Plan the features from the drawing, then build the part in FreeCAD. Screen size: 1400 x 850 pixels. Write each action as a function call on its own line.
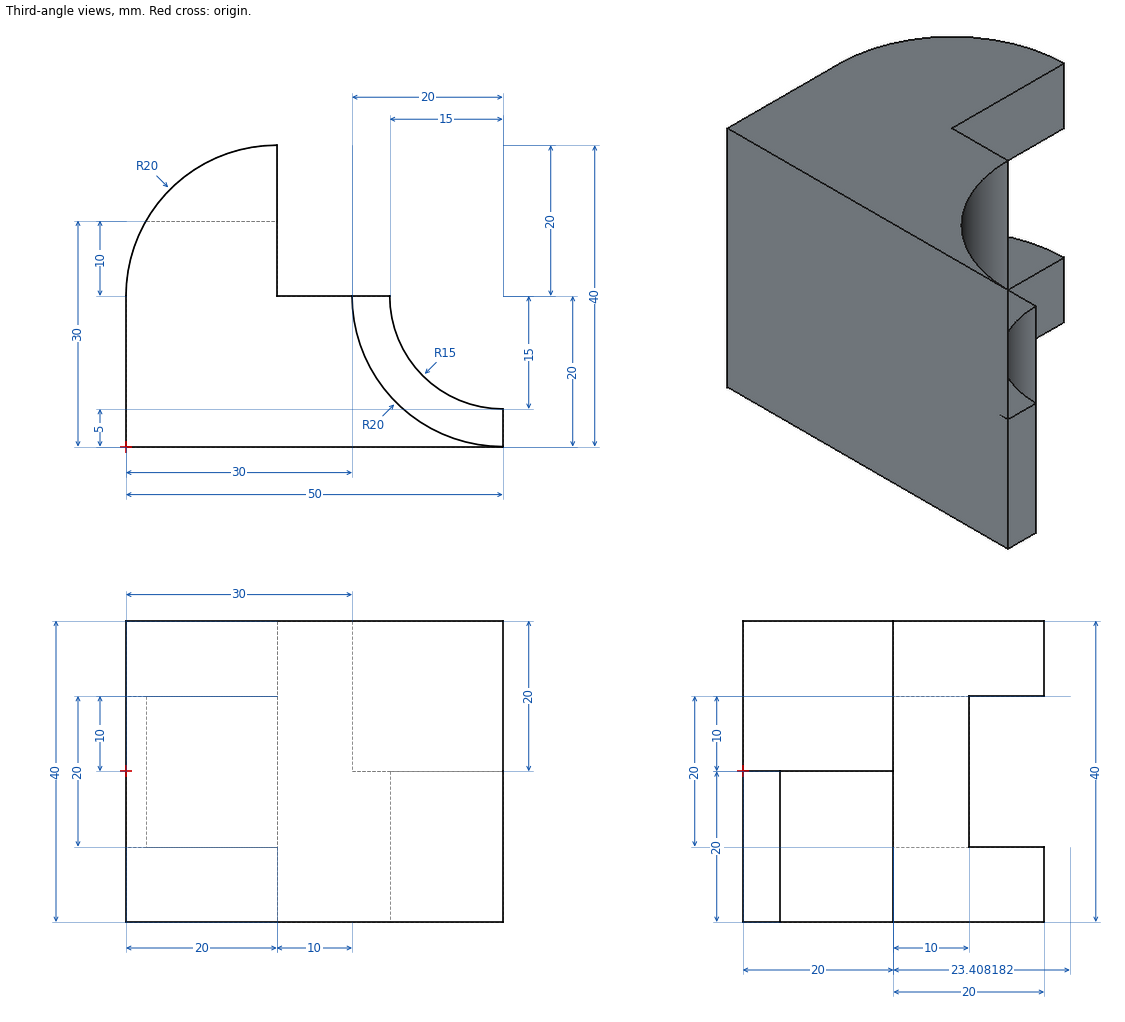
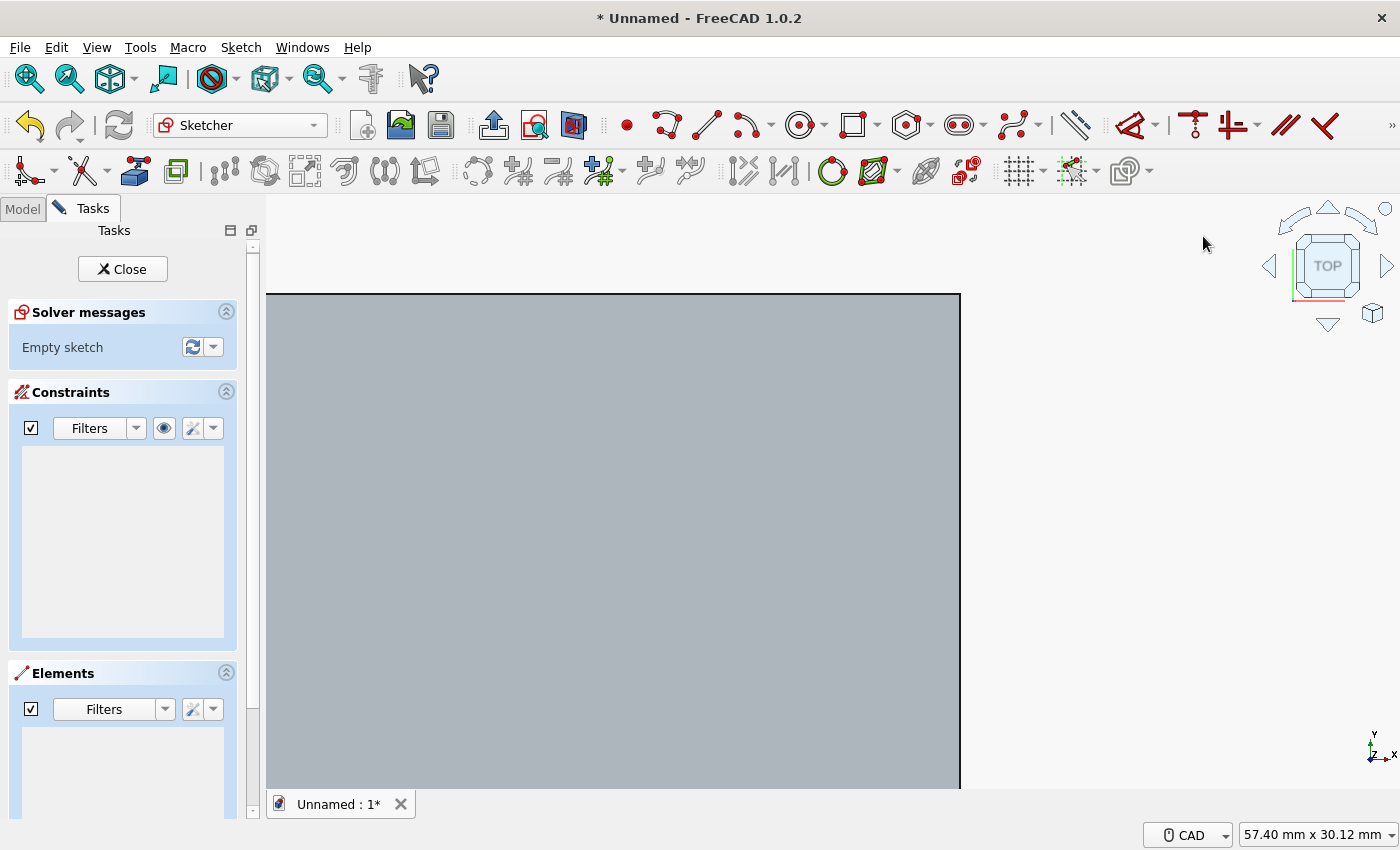
click(854, 126)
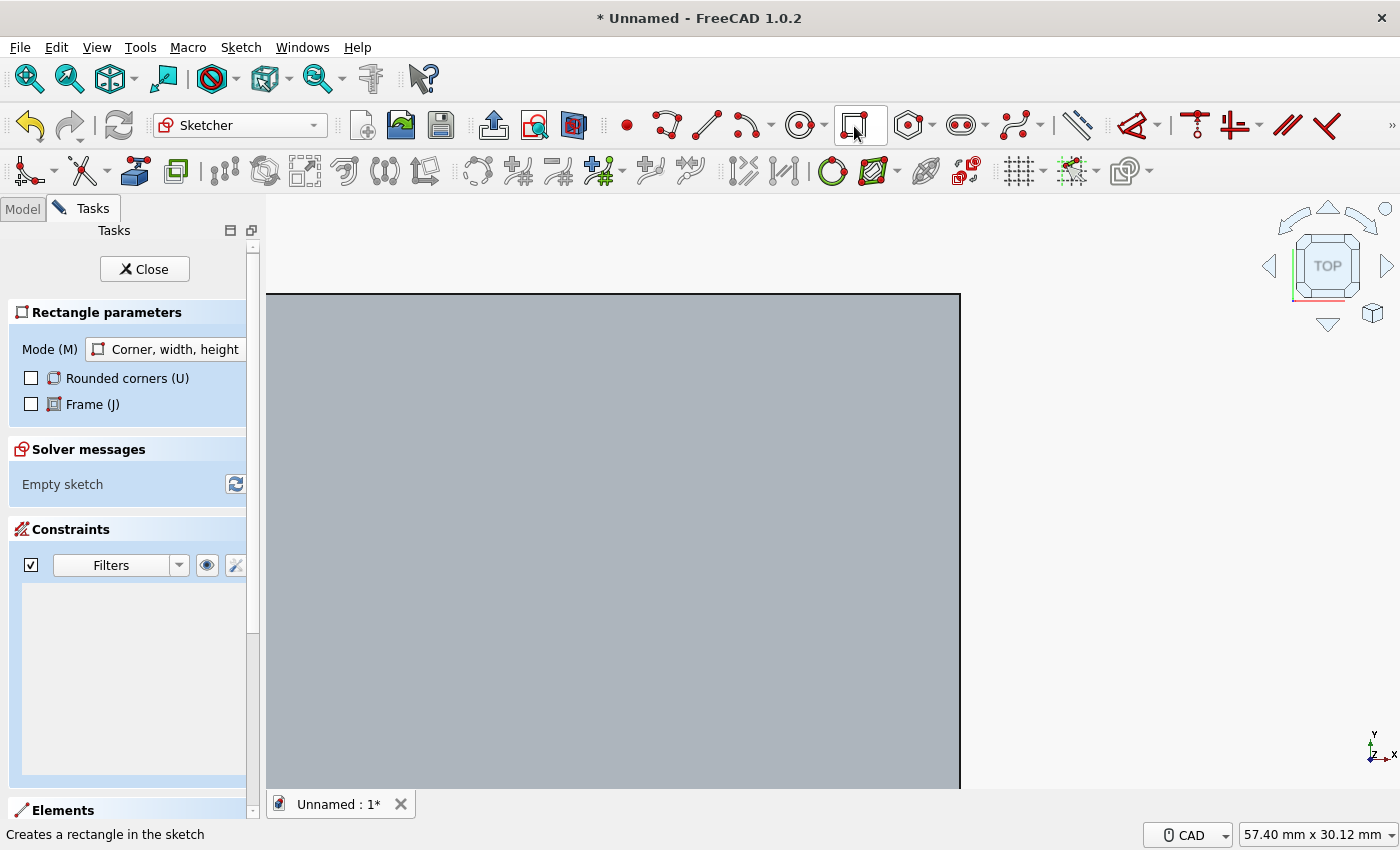
click(565, 294)
move(960, 689)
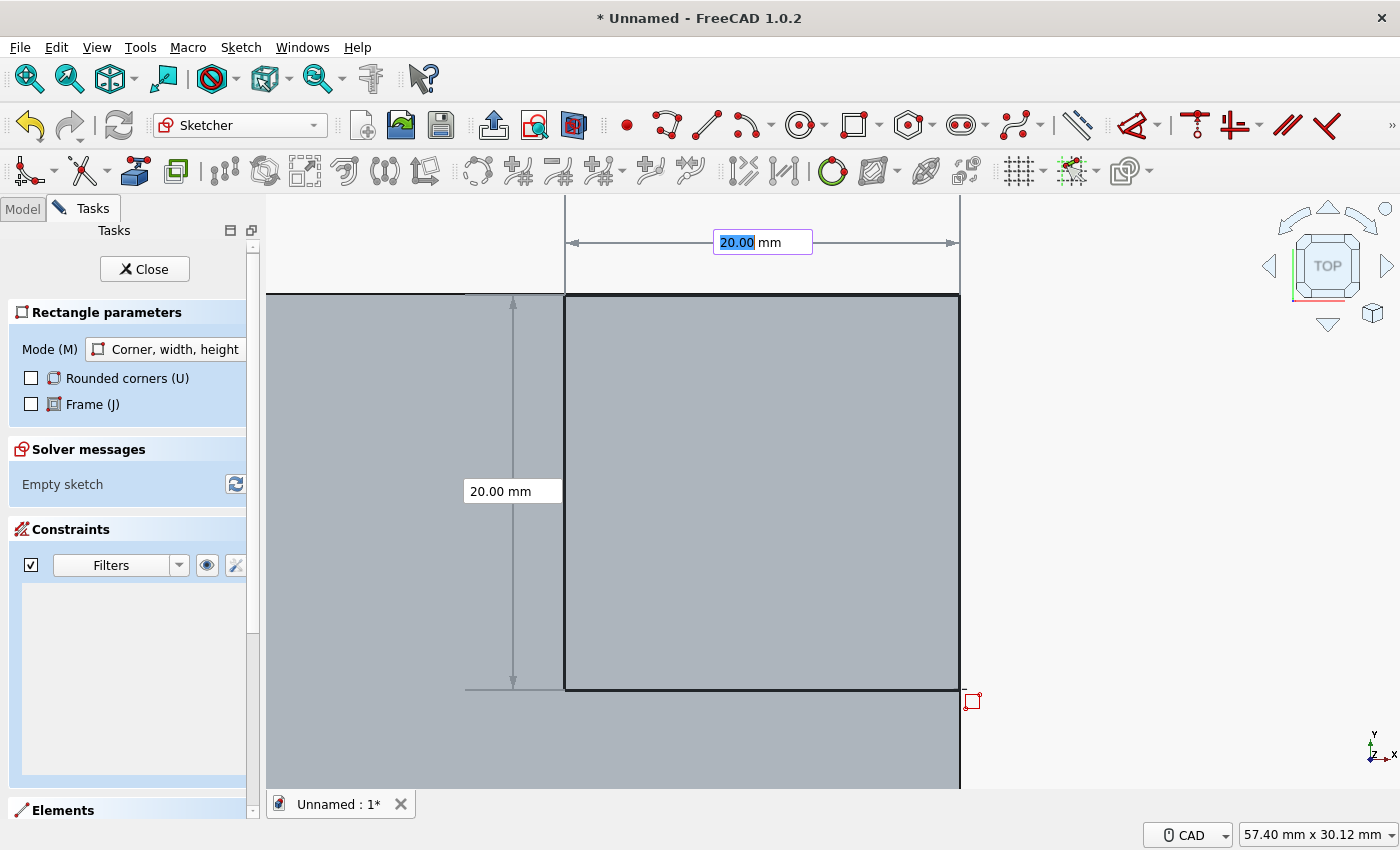
text(20)
key(Tab)
text(20)
key(Return)
key(Escape)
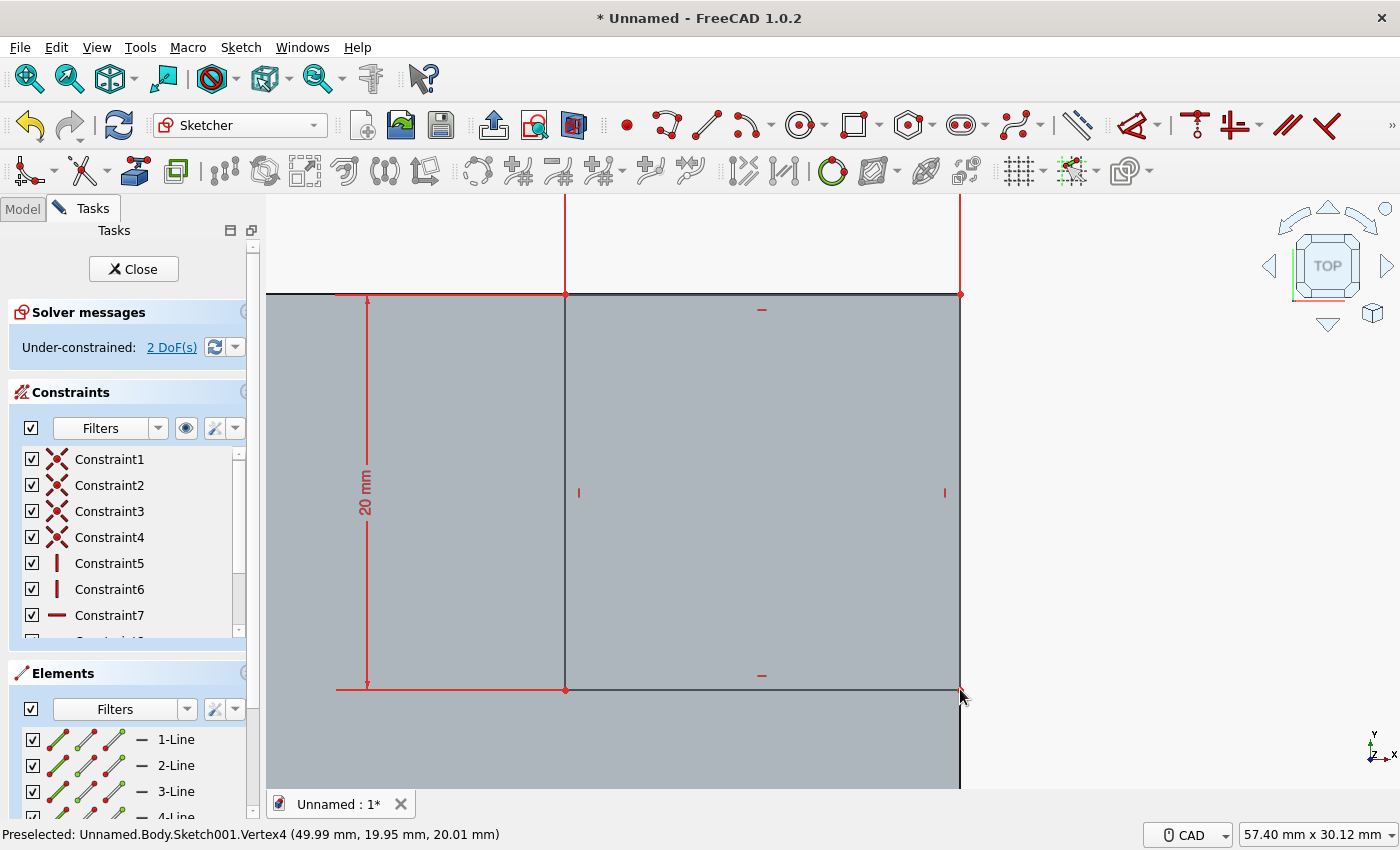
click(1132, 126)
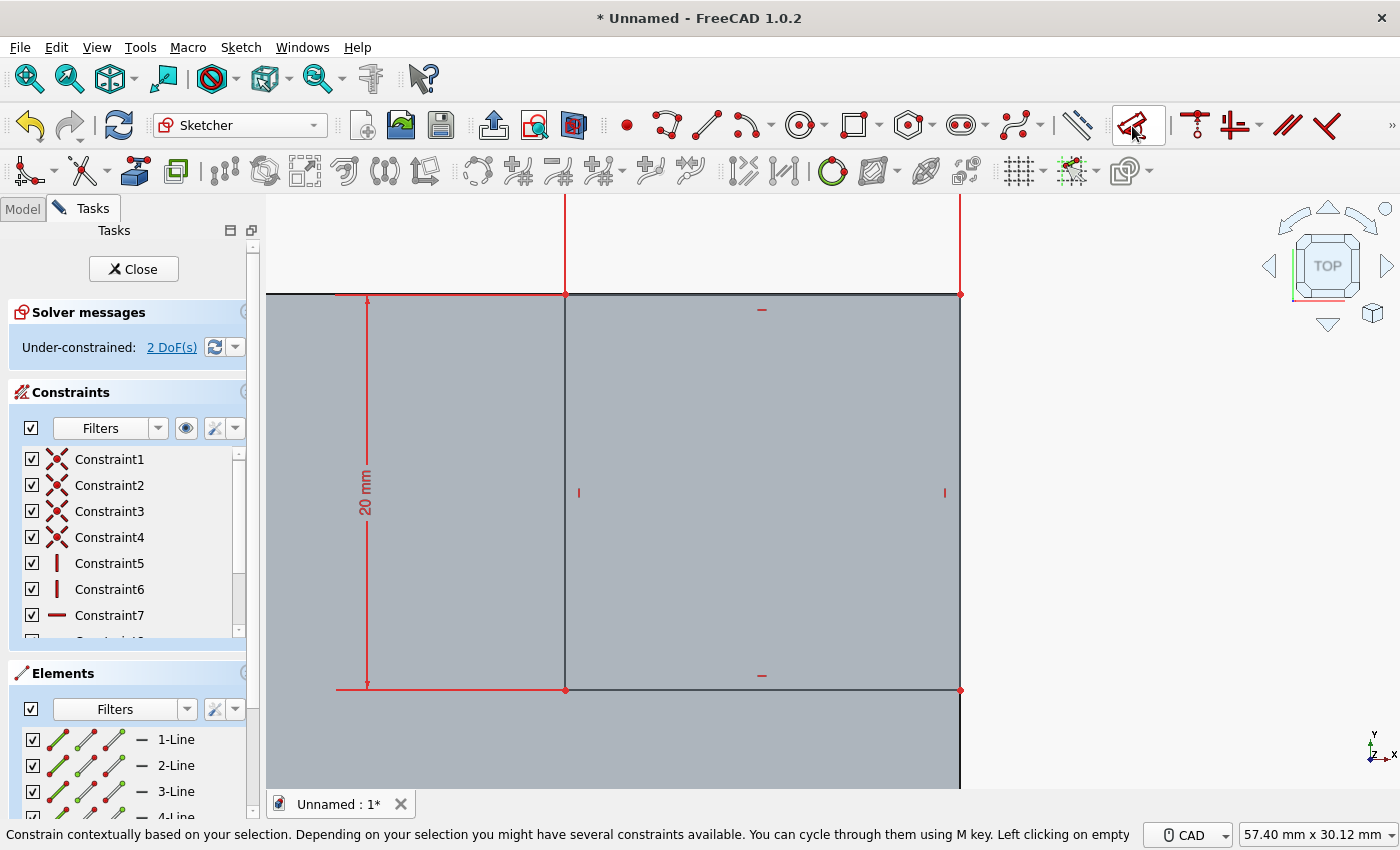
click(565, 295)
click(429, 261)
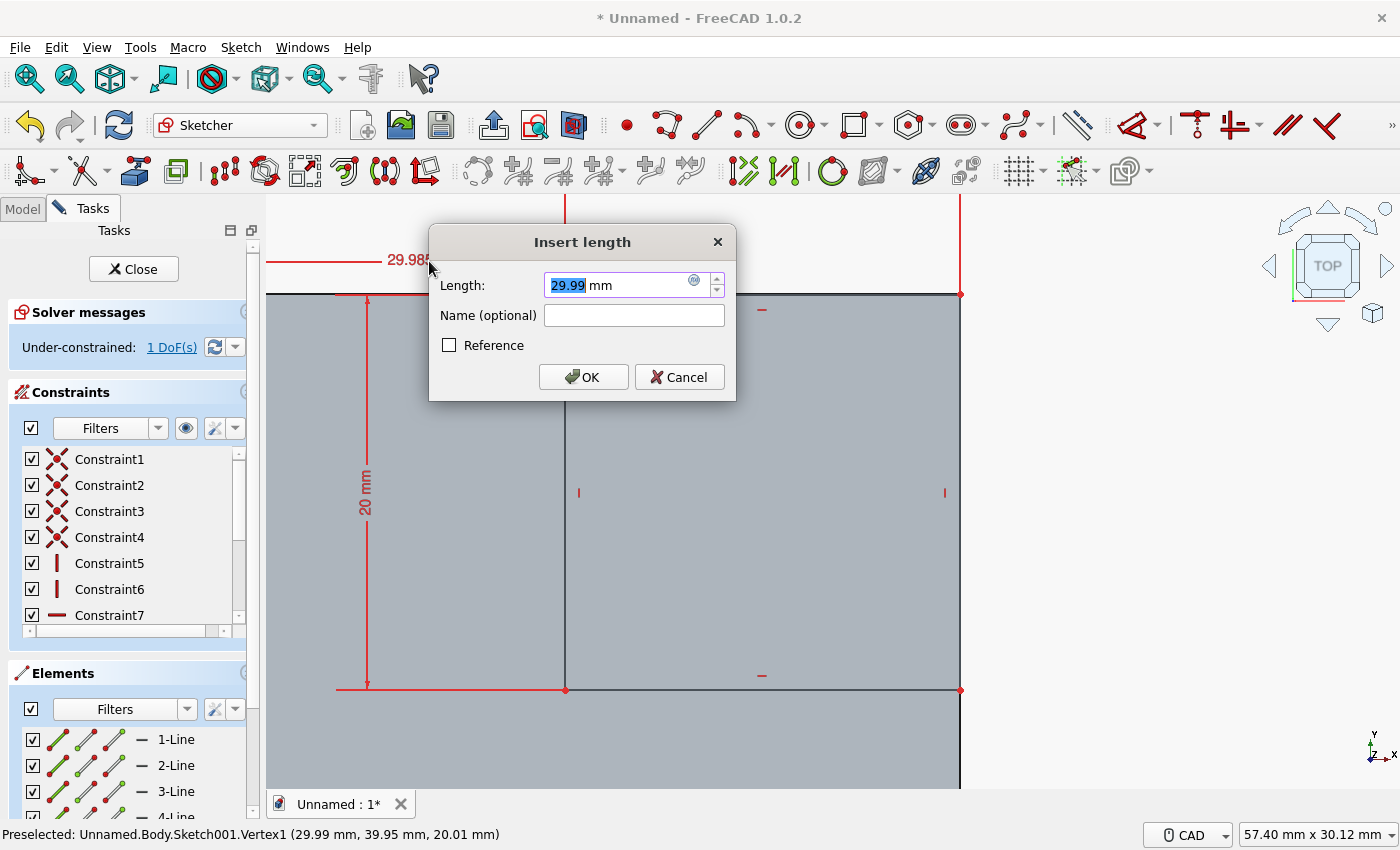
text(30)
key(Return)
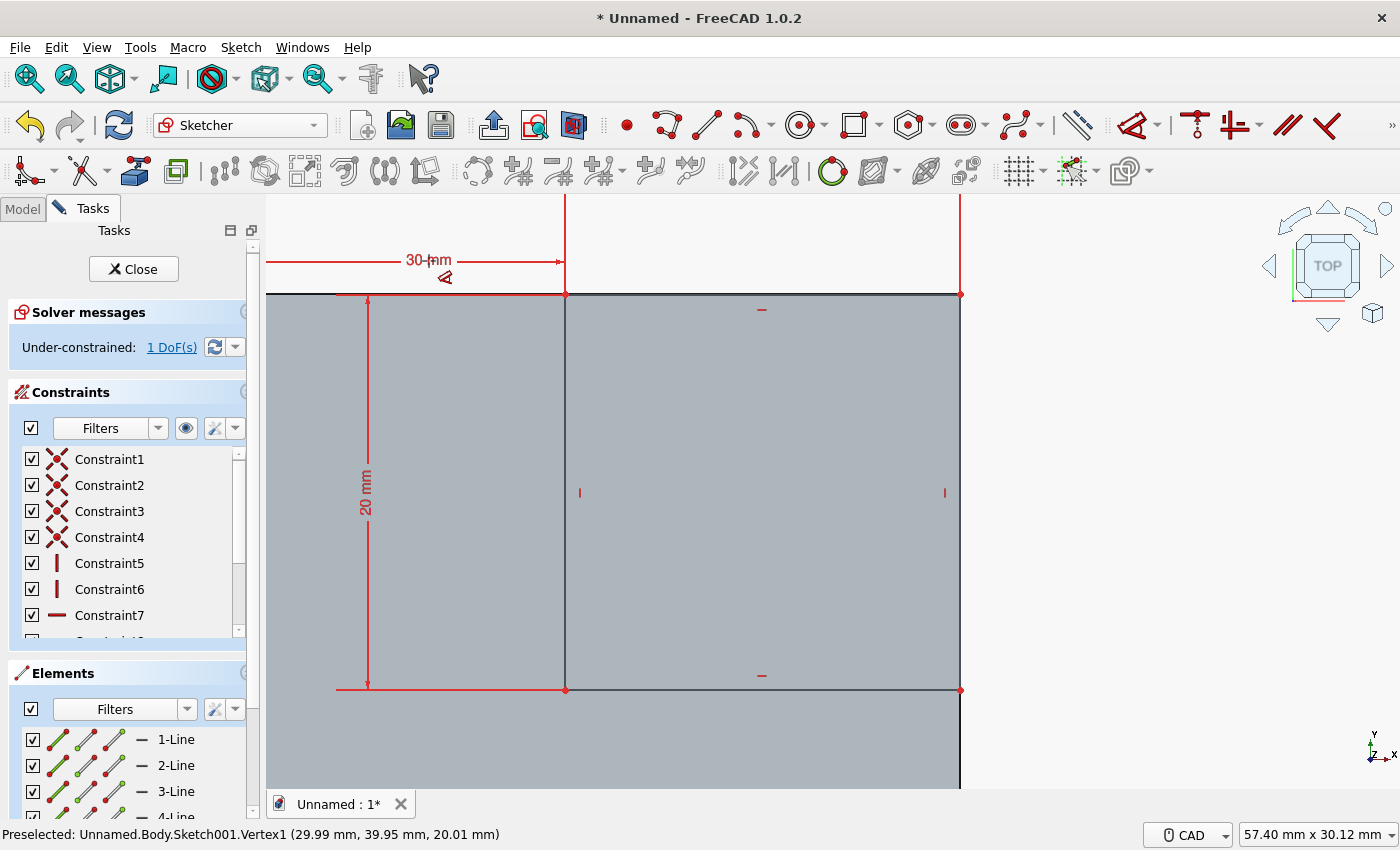
click(565, 295)
click(599, 528)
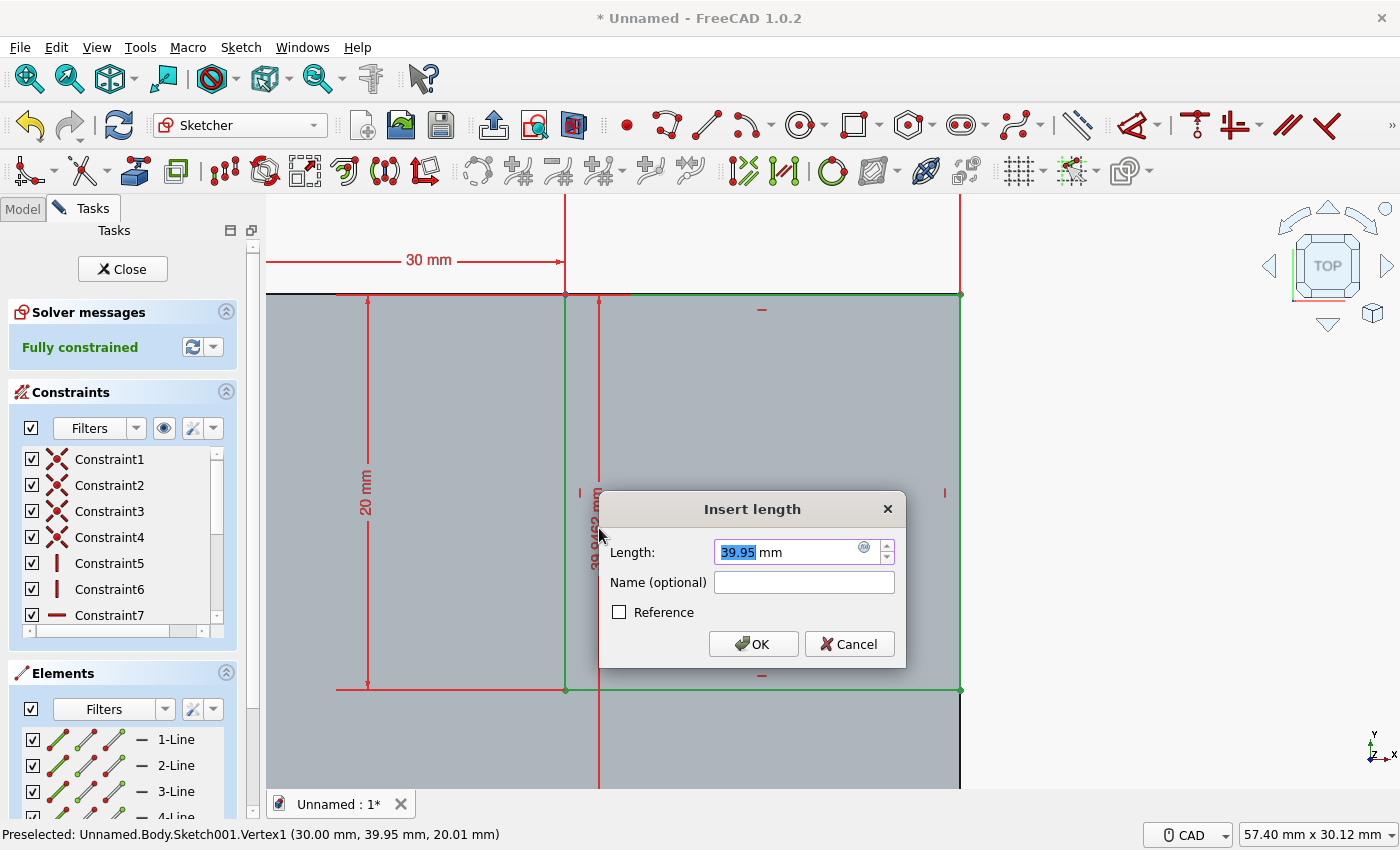
text(40)
key(Return)
key(Escape)